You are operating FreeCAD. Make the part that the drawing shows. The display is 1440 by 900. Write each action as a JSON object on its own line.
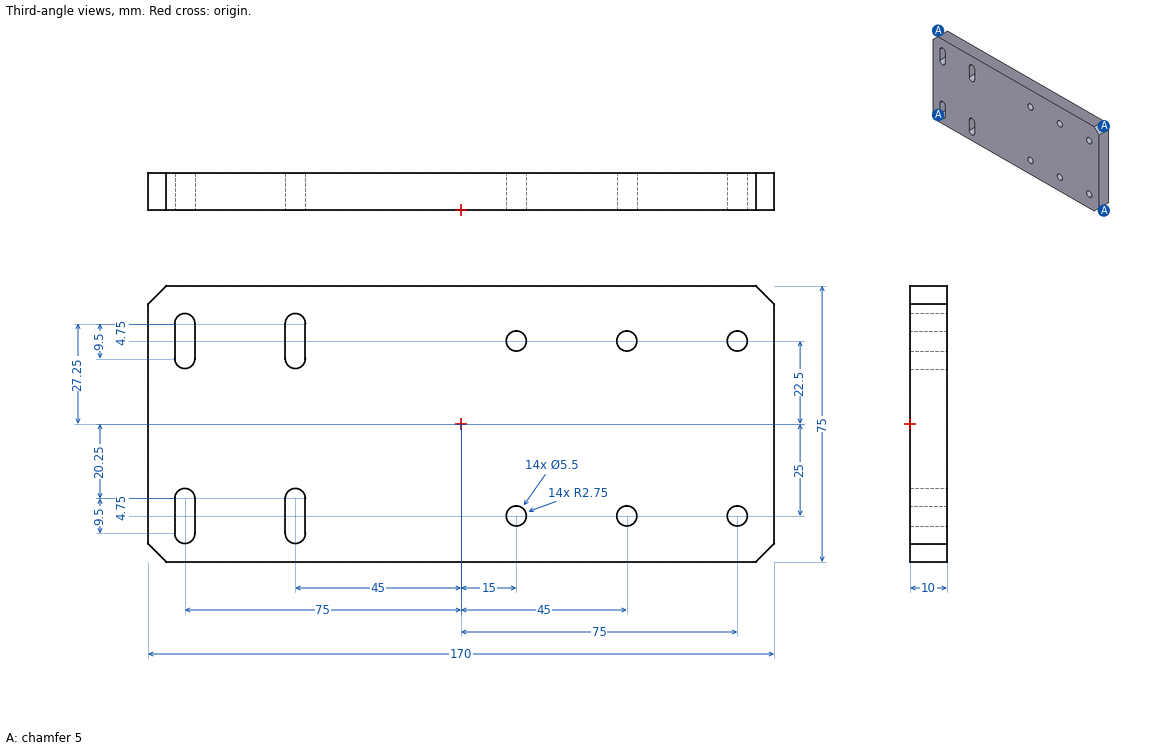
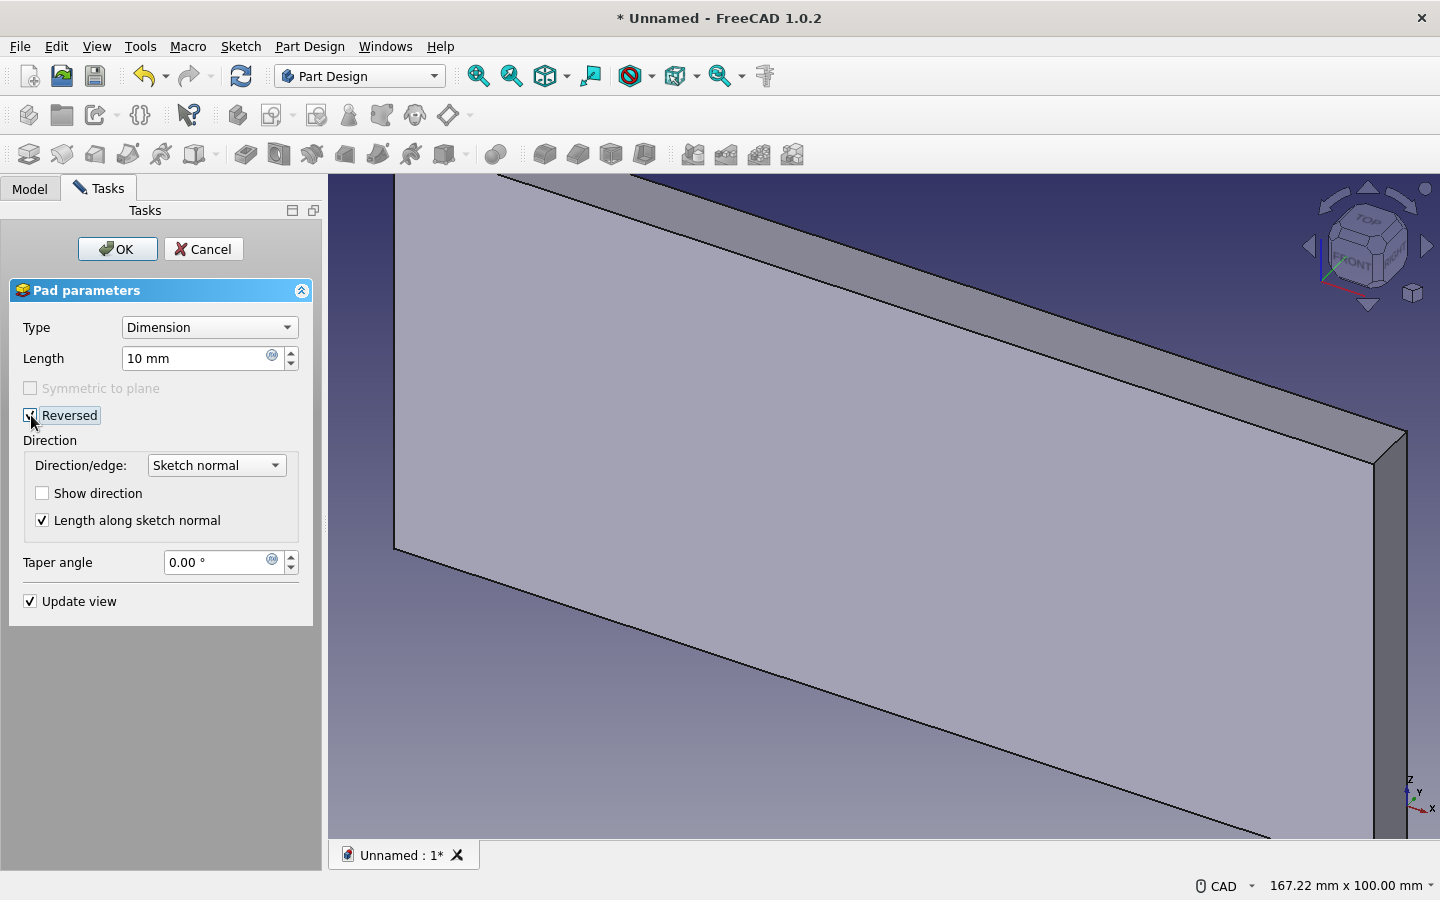
{"action": "left_click", "coordinate": [118, 249]}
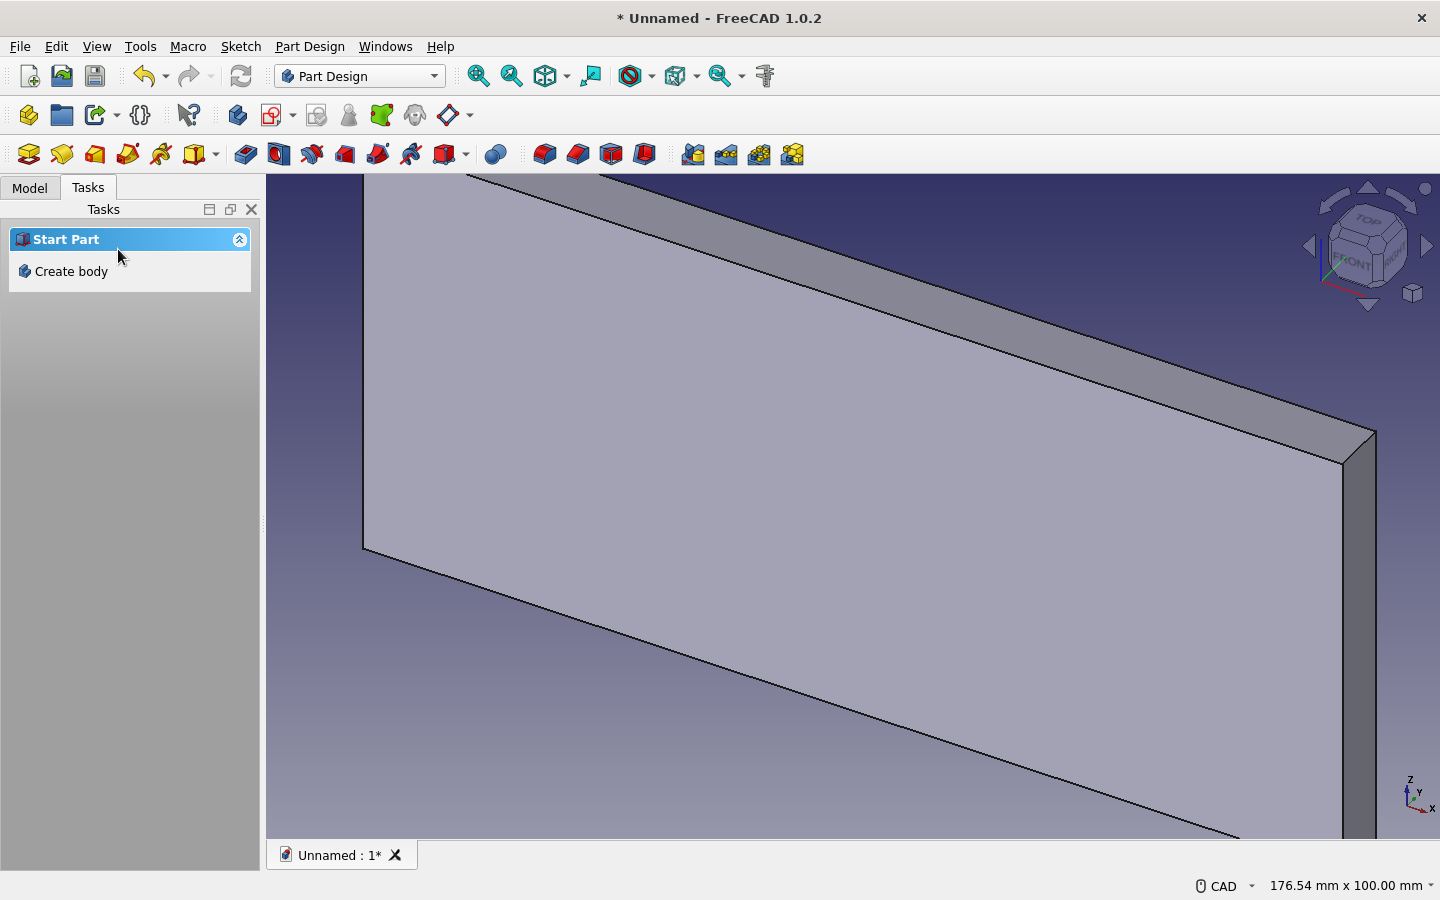
{"action": "key", "text": "v f"}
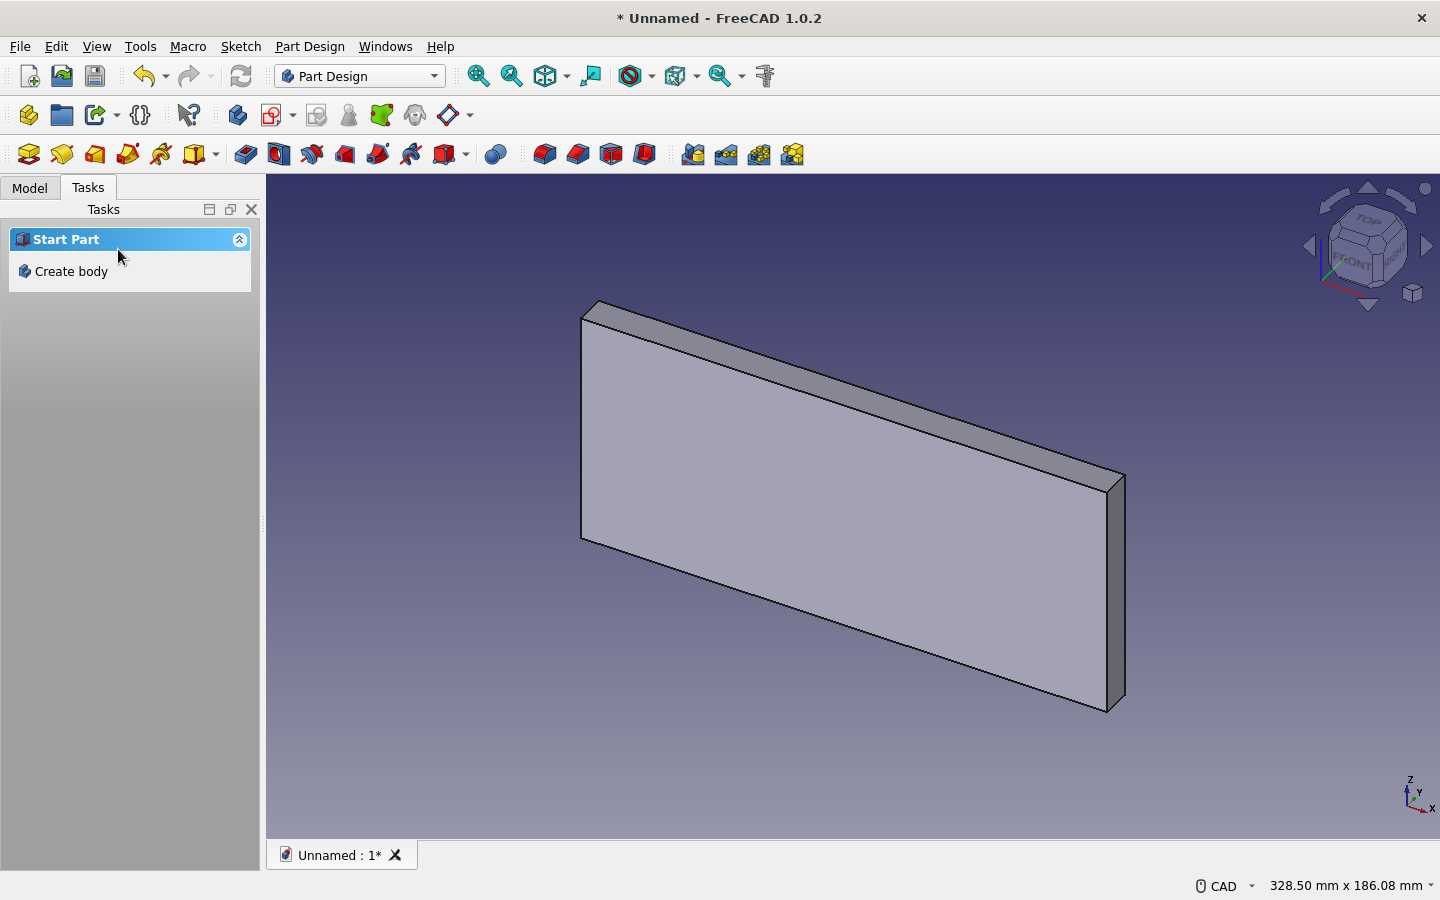
{"action": "left_click", "coordinate": [1116, 483]}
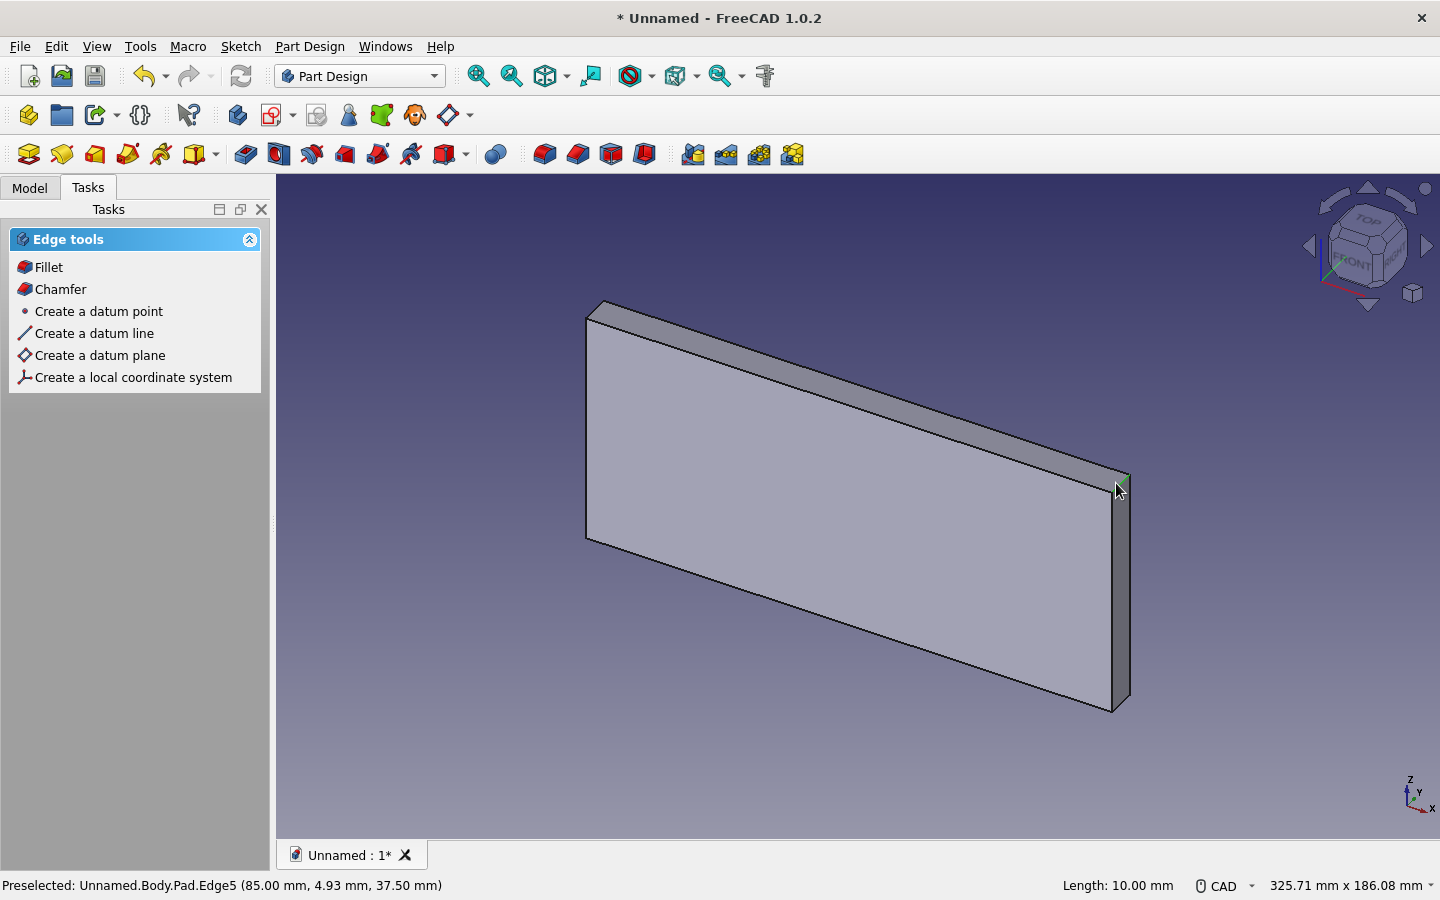
{"action": "key", "text": "0"}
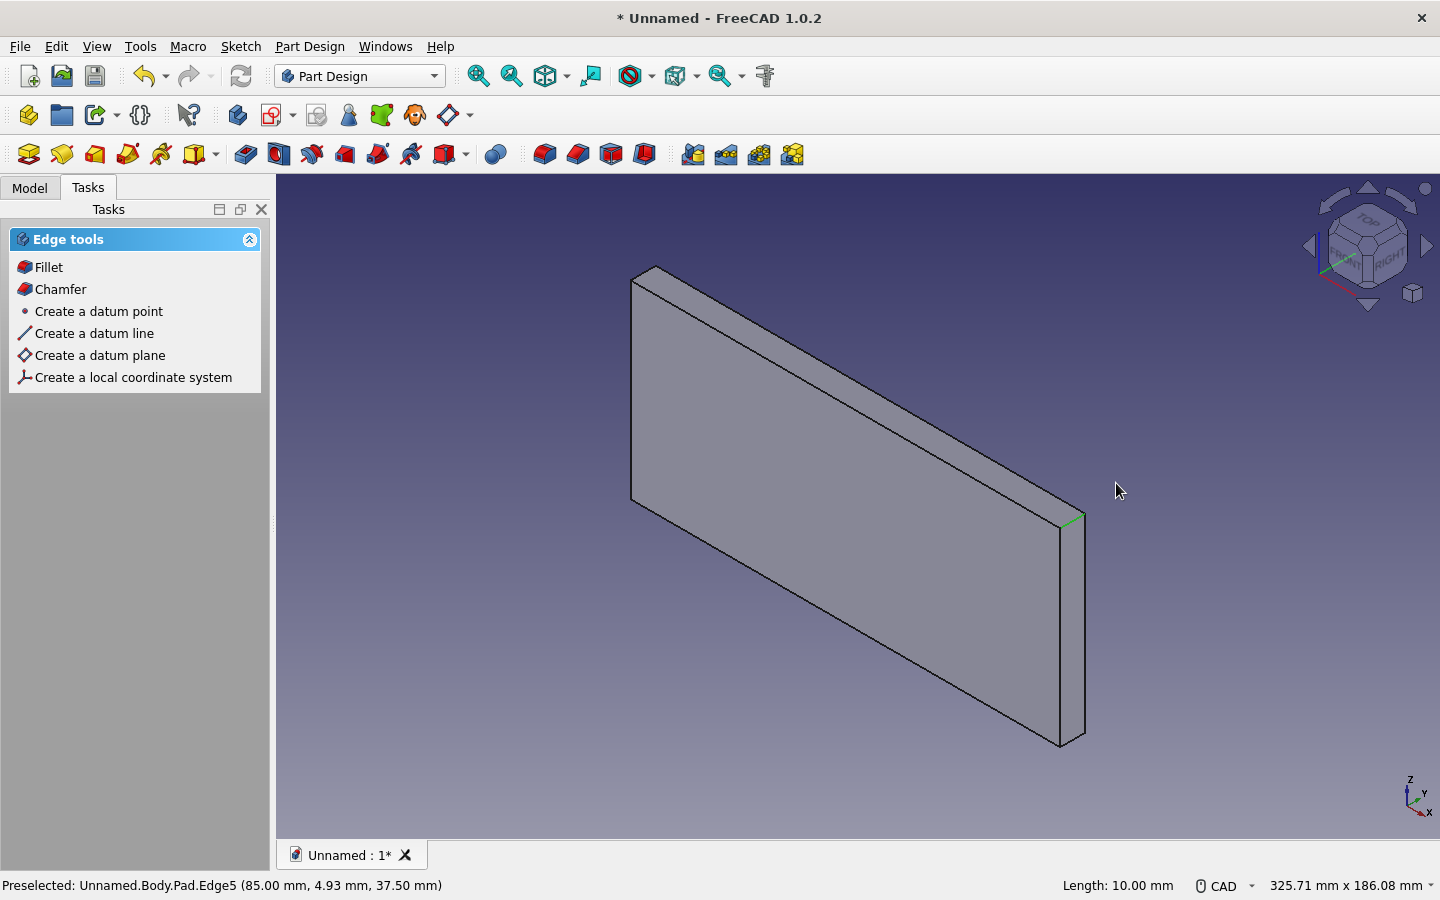
{"action": "key", "text": "2"}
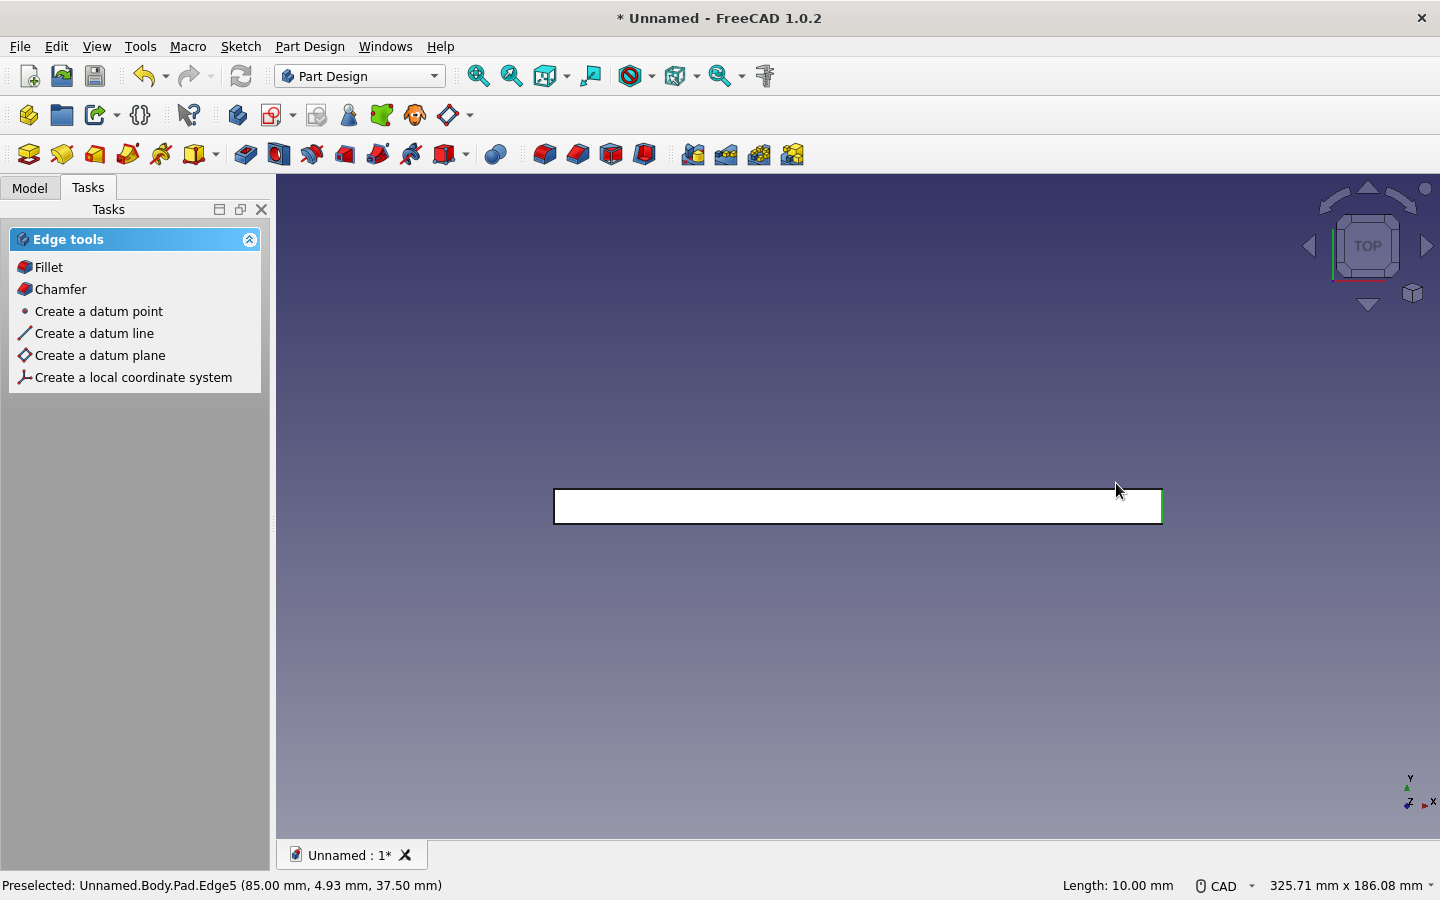
{"action": "left_click", "coordinate": [554, 506], "text": "ctrl"}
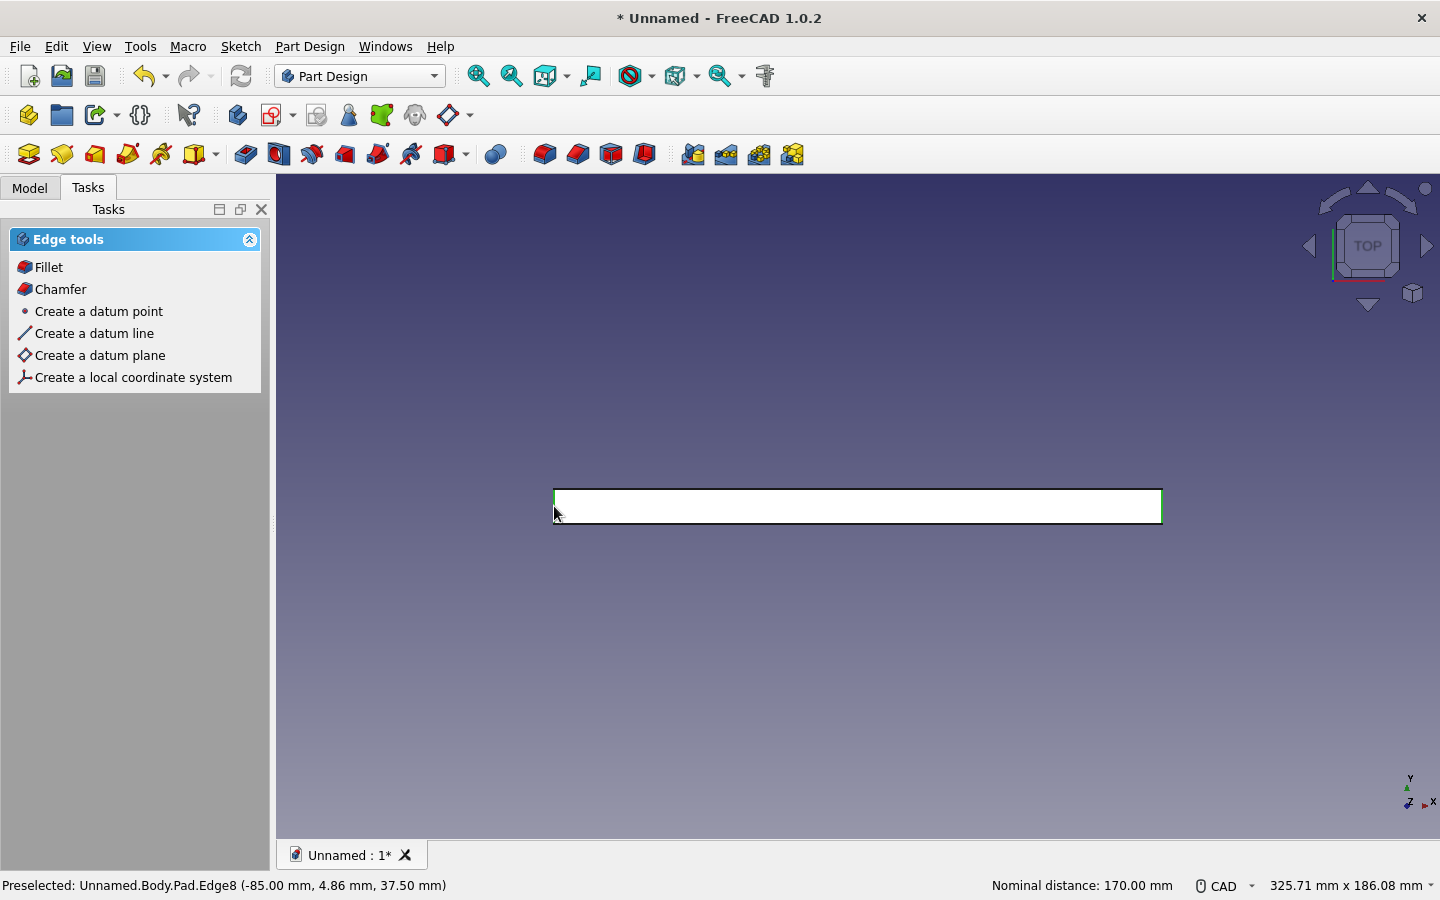
{"action": "key", "text": "1"}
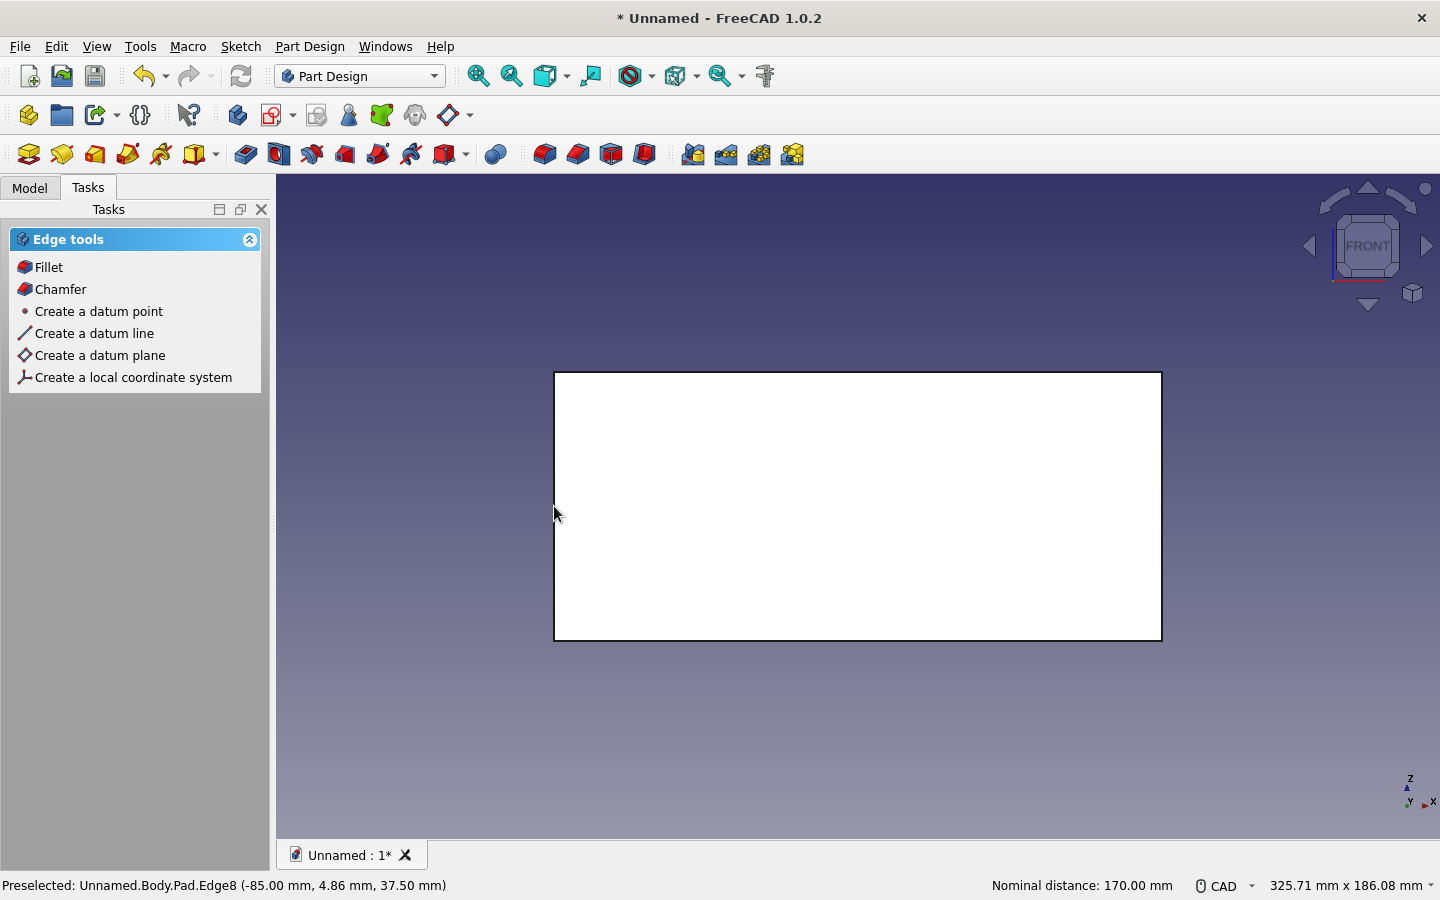
{"action": "key", "text": "3"}